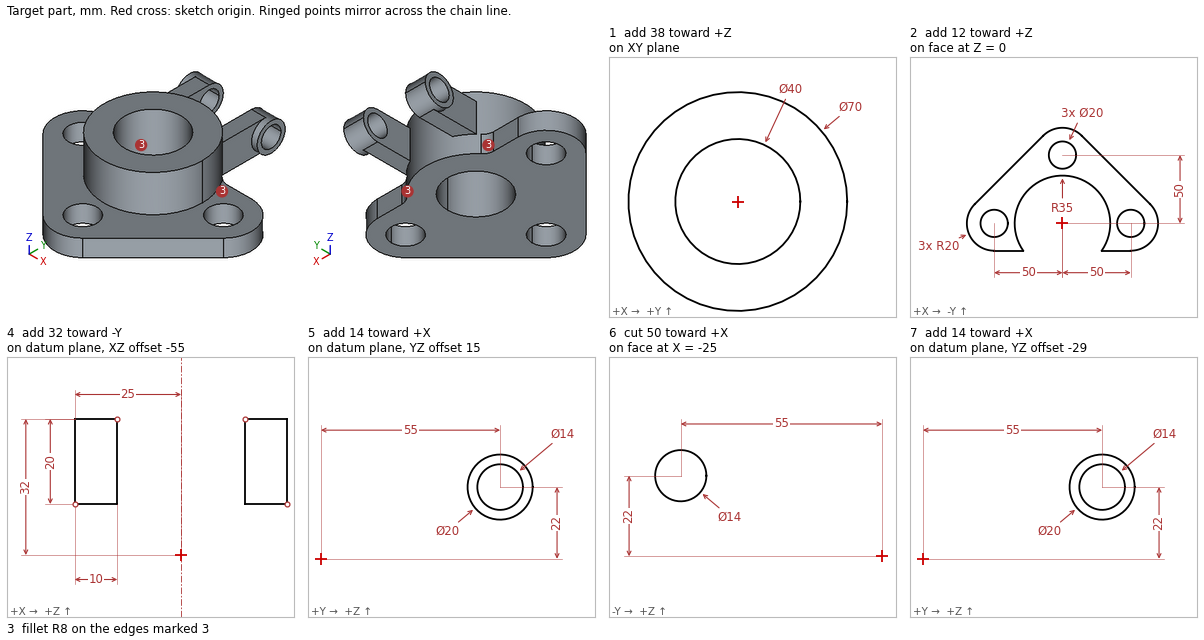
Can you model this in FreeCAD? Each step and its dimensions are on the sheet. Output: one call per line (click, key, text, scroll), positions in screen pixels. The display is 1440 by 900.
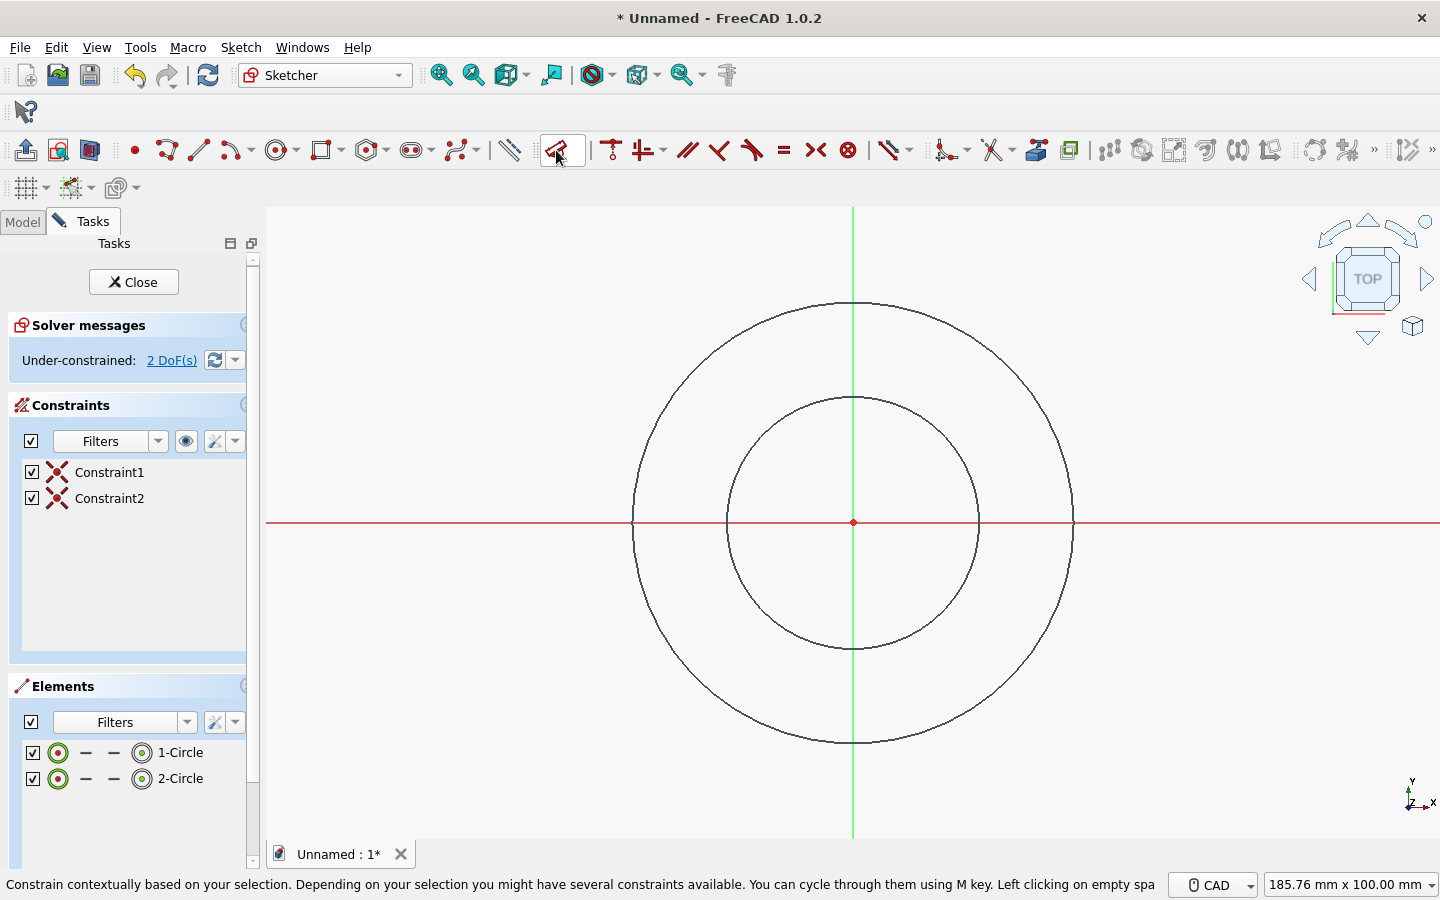
click(1009, 367)
click(1032, 344)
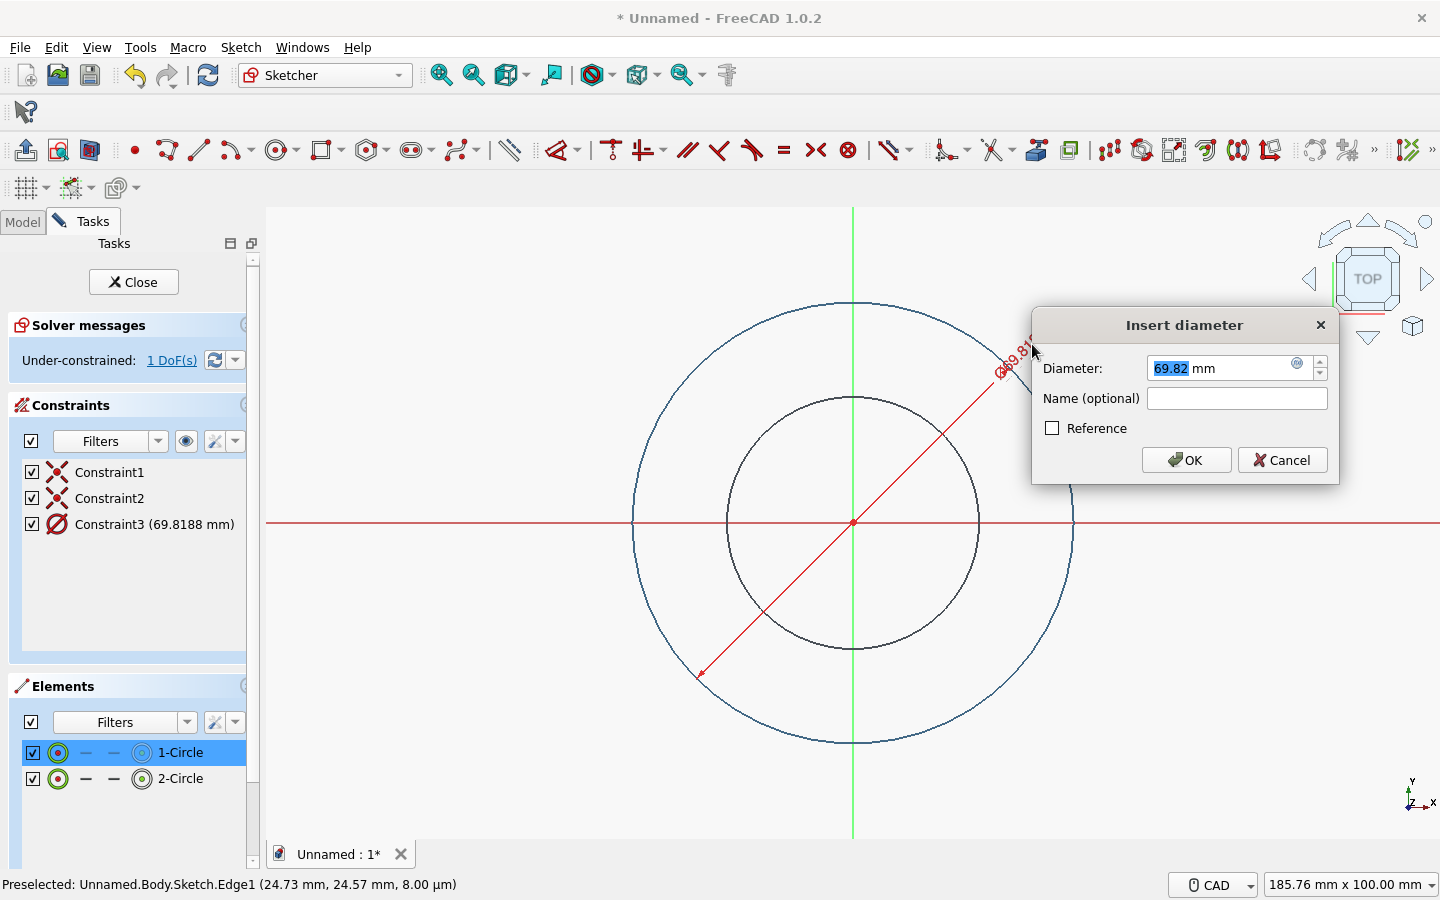
text(70)
key(Return)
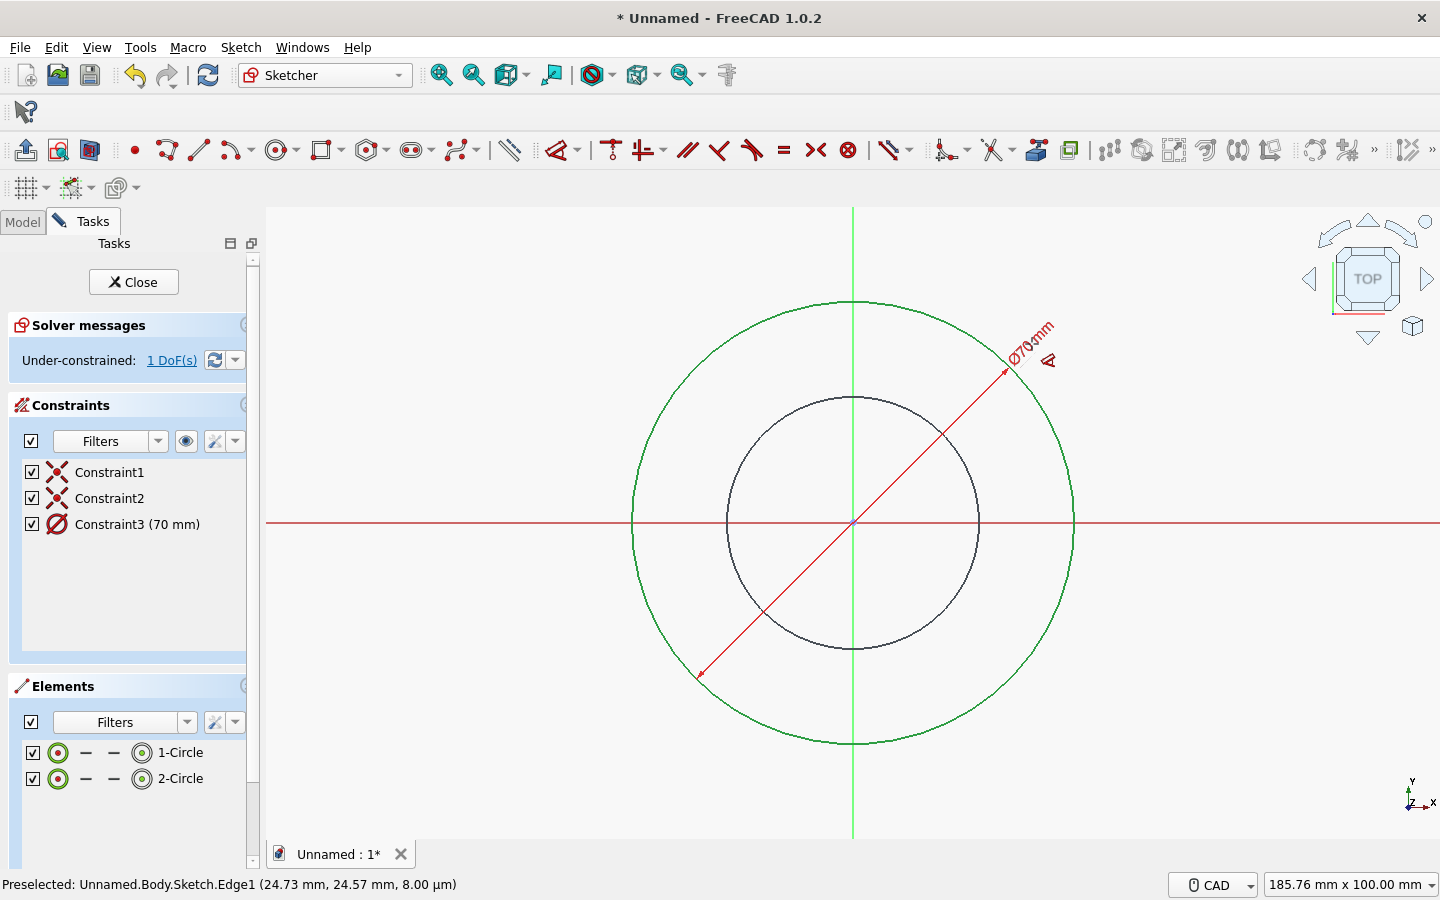
click(942, 434)
click(965, 411)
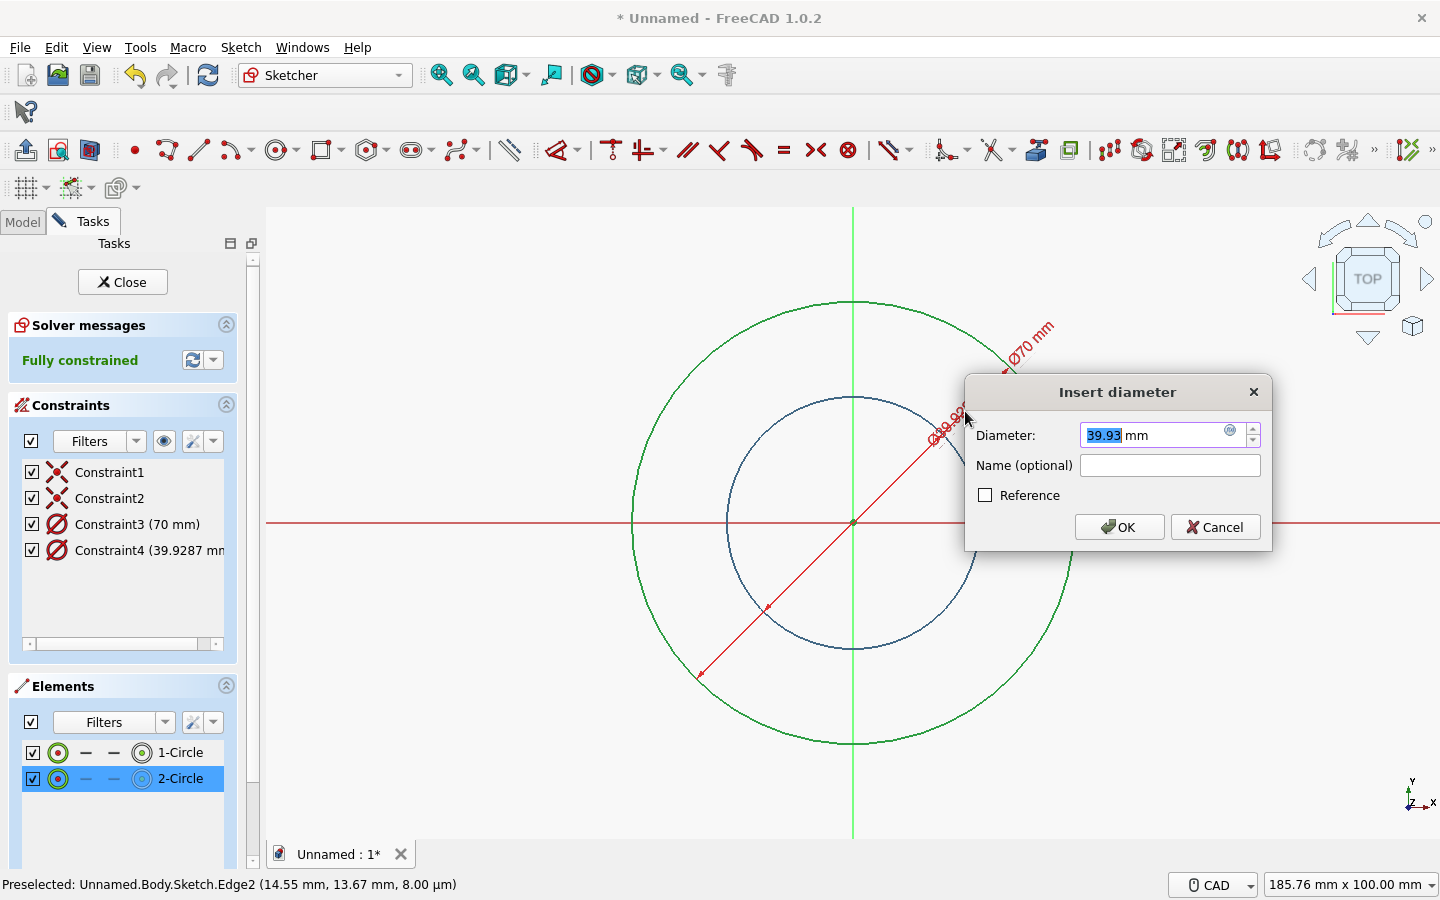
text(40)
key(Return)
key(Escape)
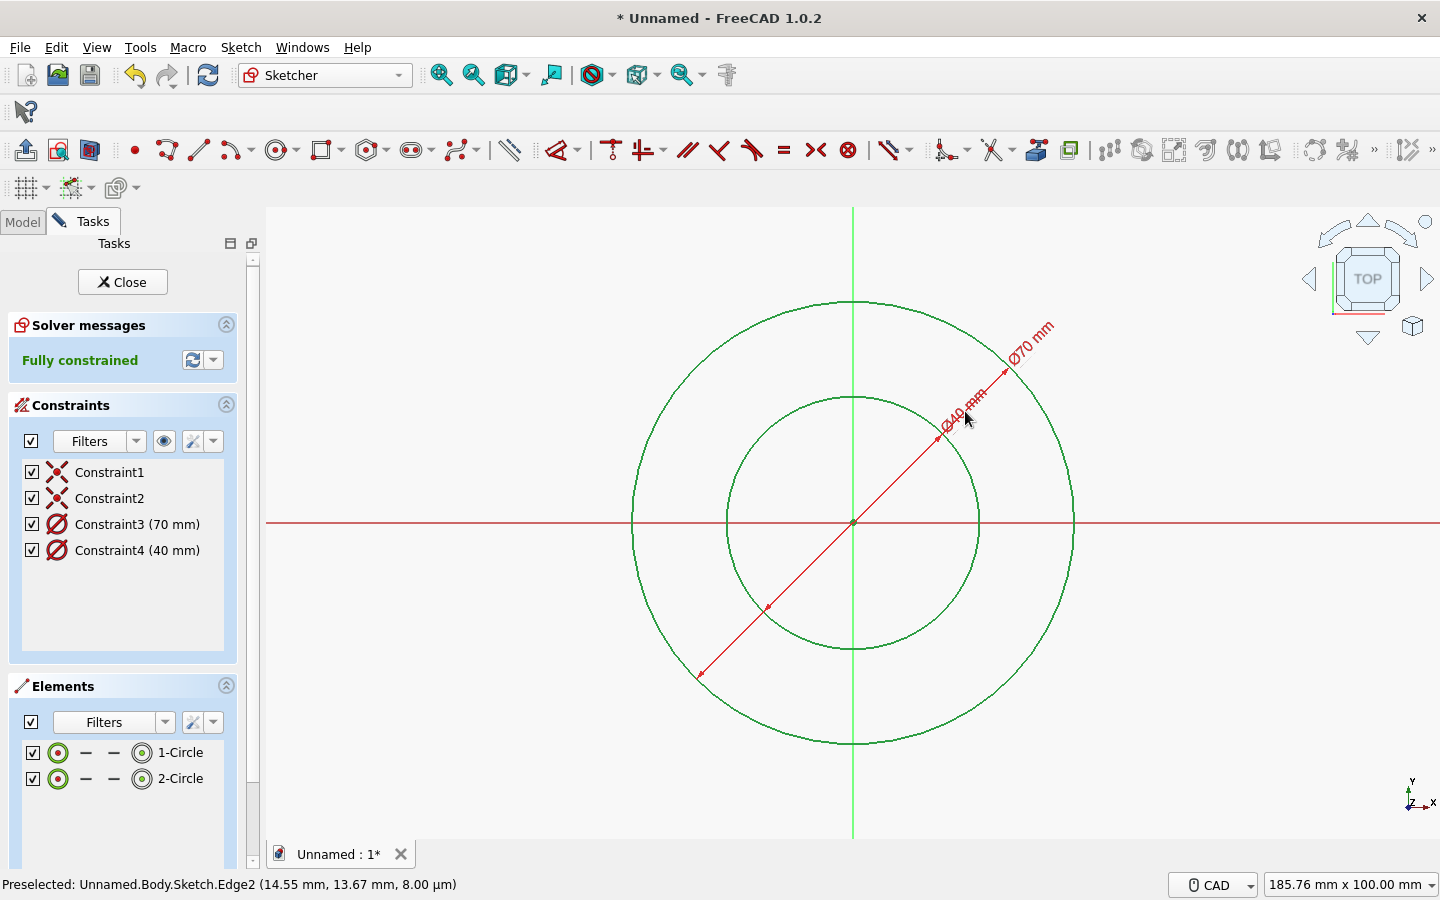
click(123, 282)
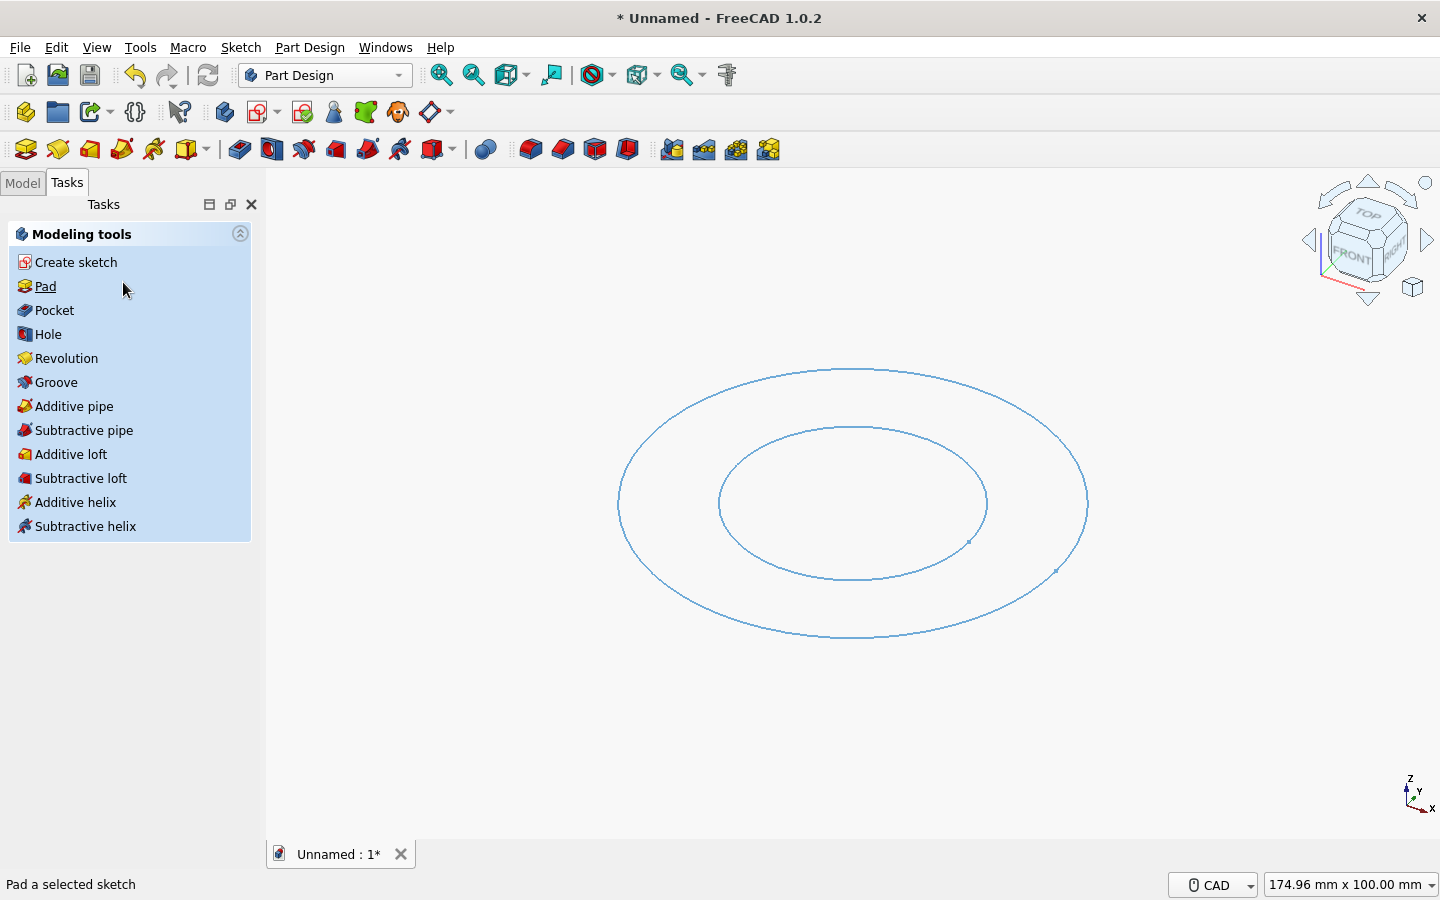
click(26, 150)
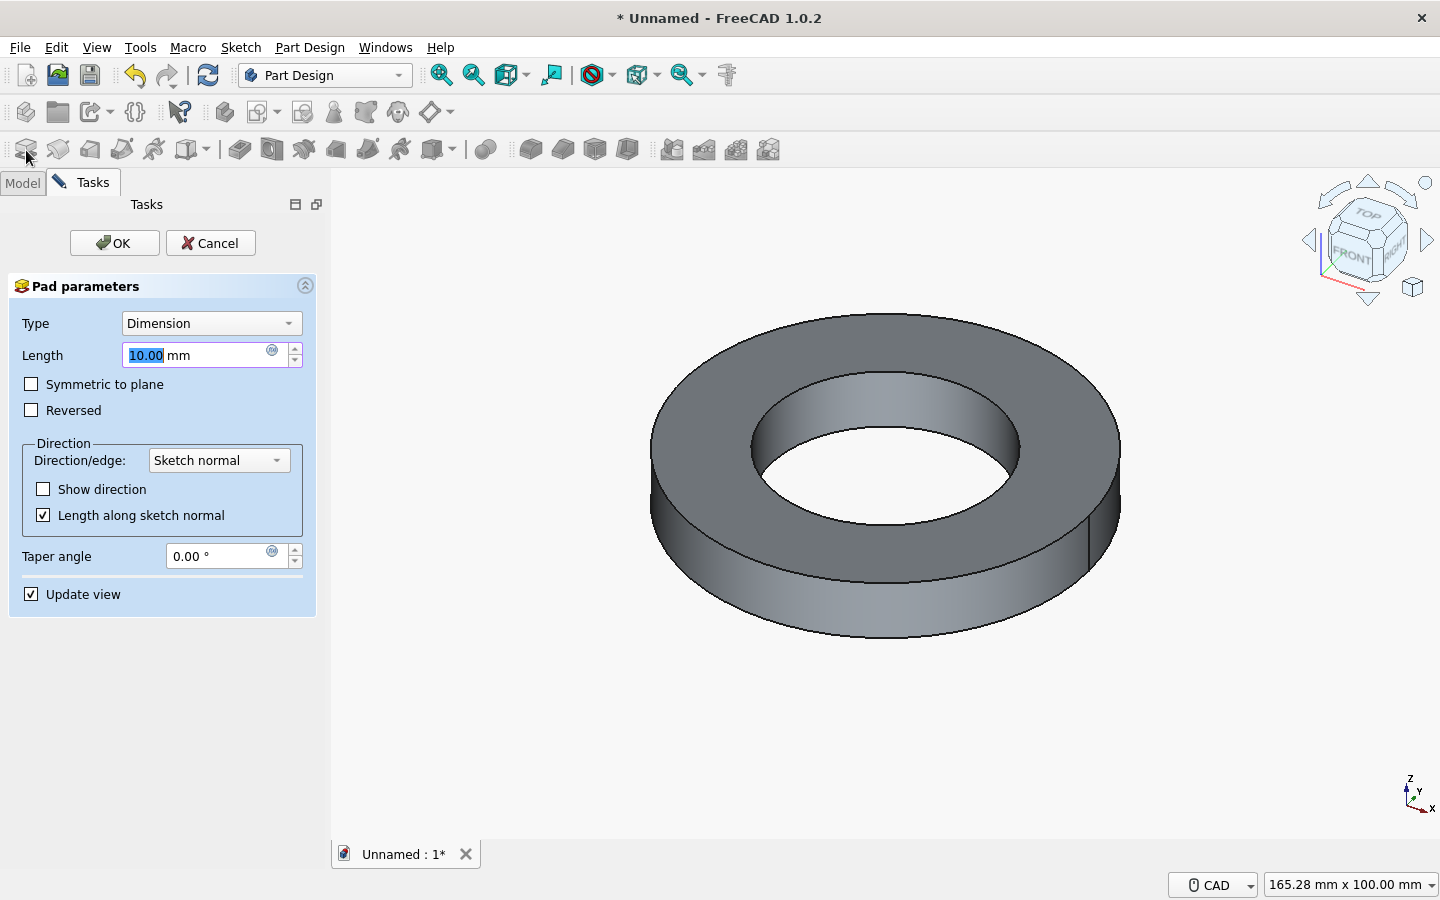
text(38)
key(Tab)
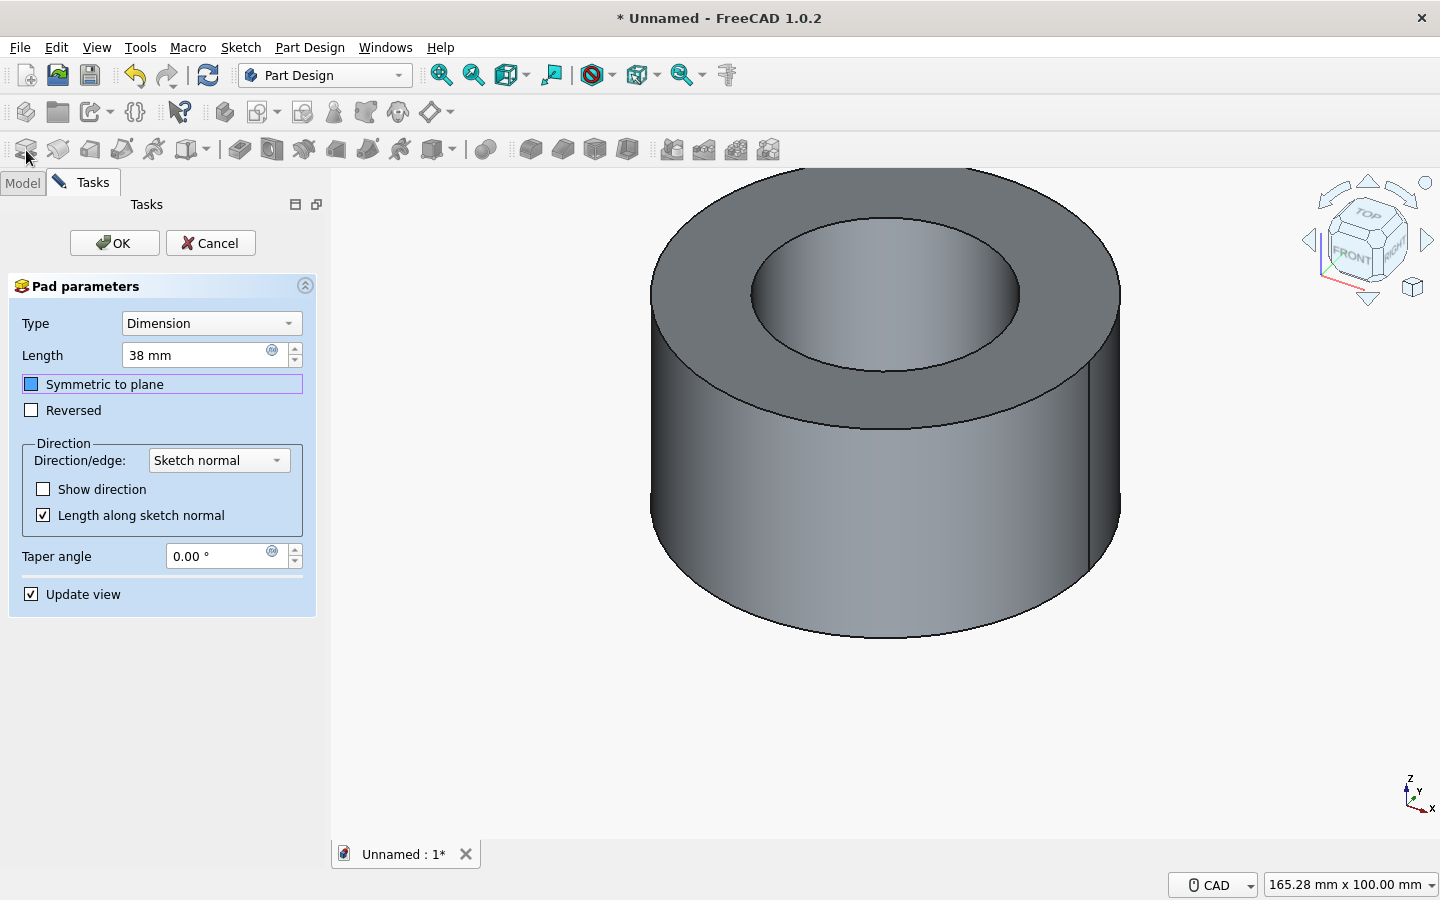
click(115, 243)